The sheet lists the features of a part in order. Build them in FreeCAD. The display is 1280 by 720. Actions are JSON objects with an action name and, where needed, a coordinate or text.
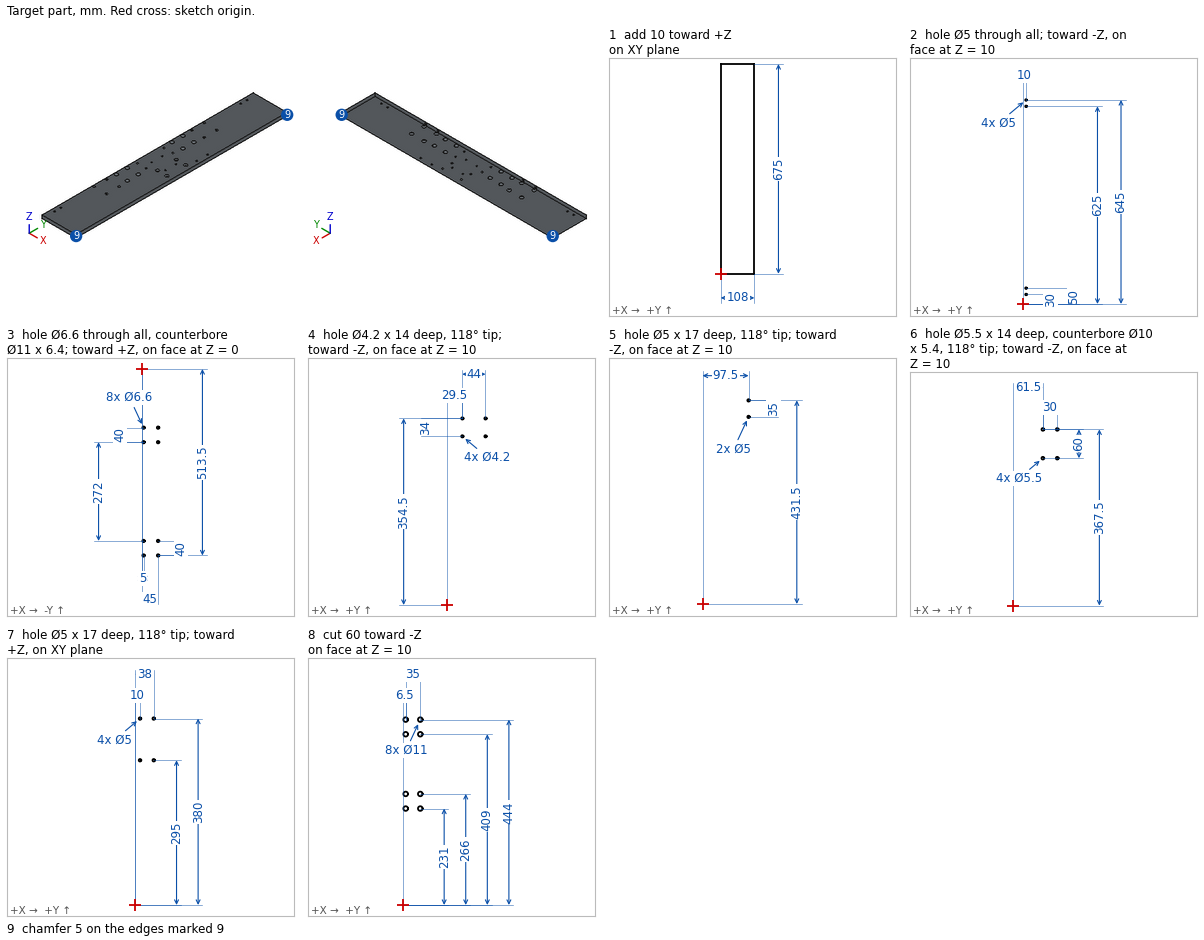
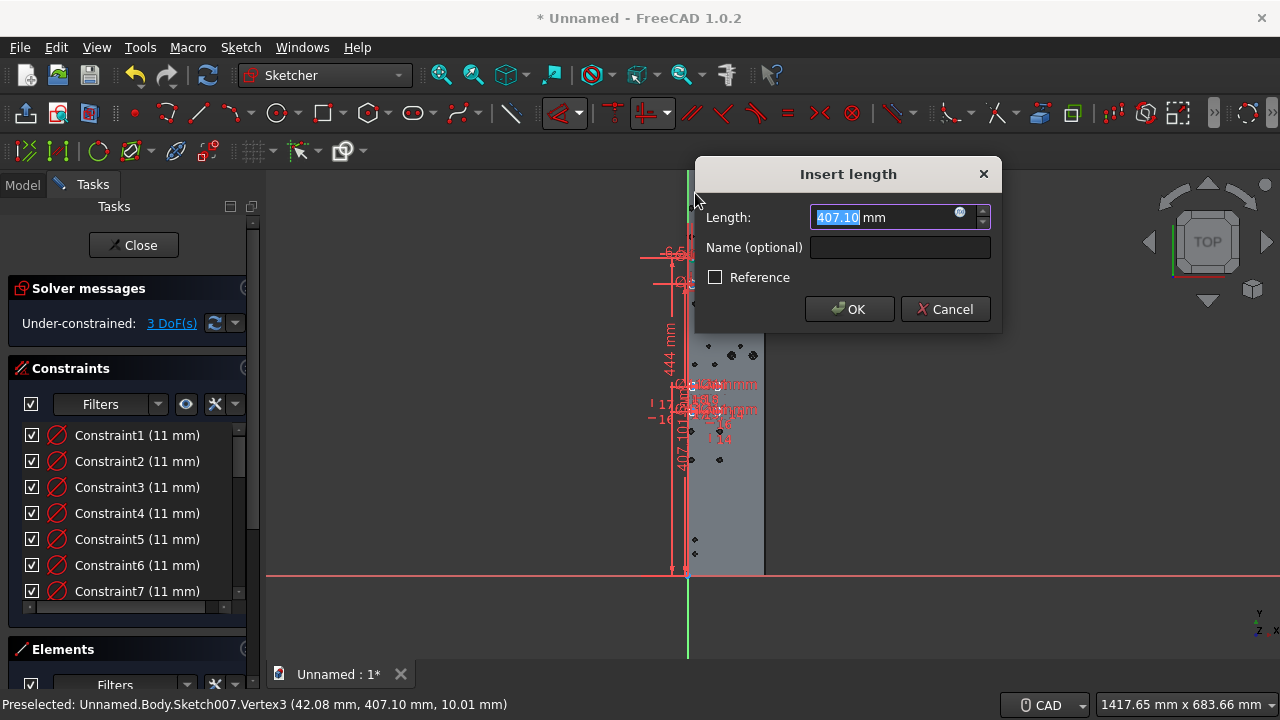
{"action": "type", "text": "409"}
{"action": "key", "text": "Return"}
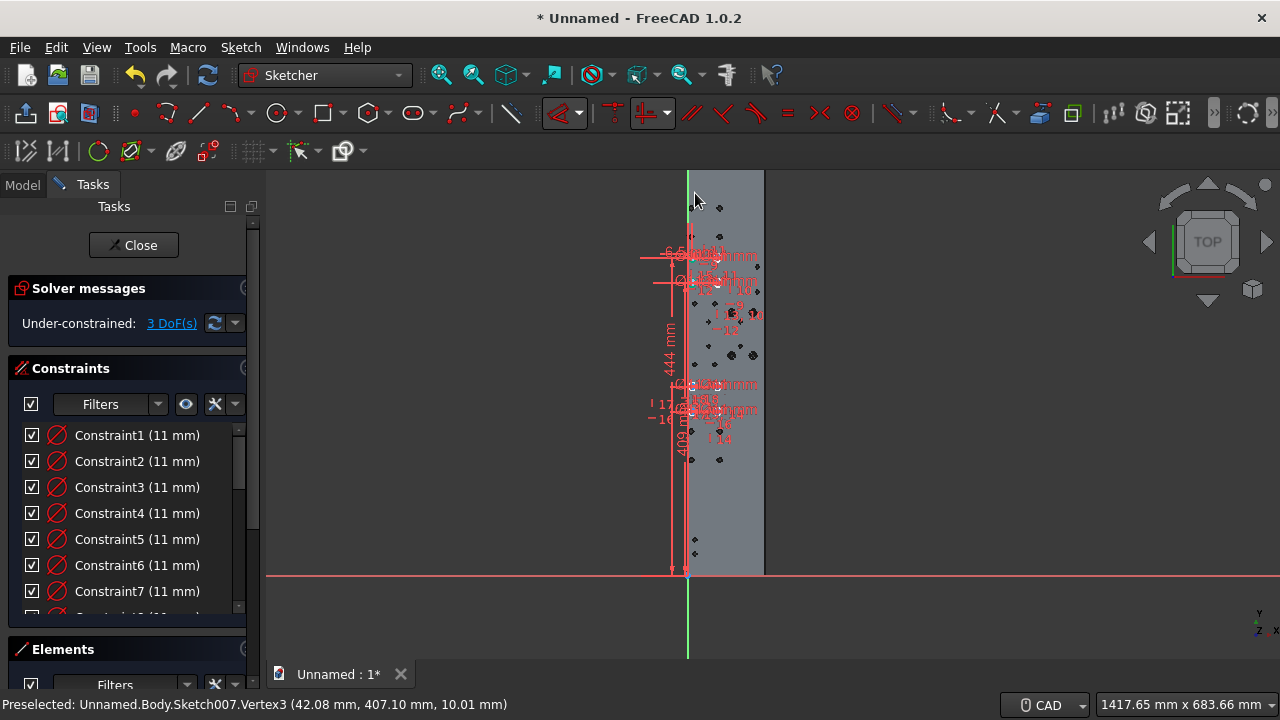
{"action": "left_click", "coordinate": [718, 387]}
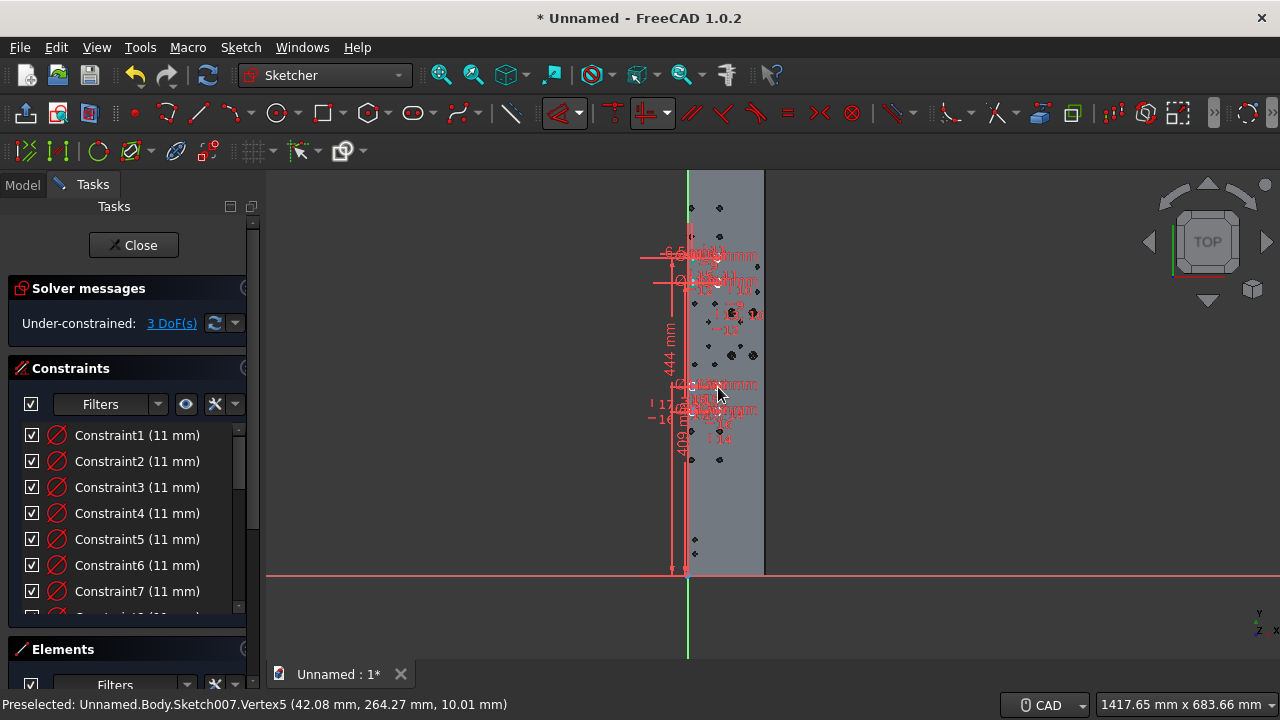
{"action": "left_click", "coordinate": [582, 114]}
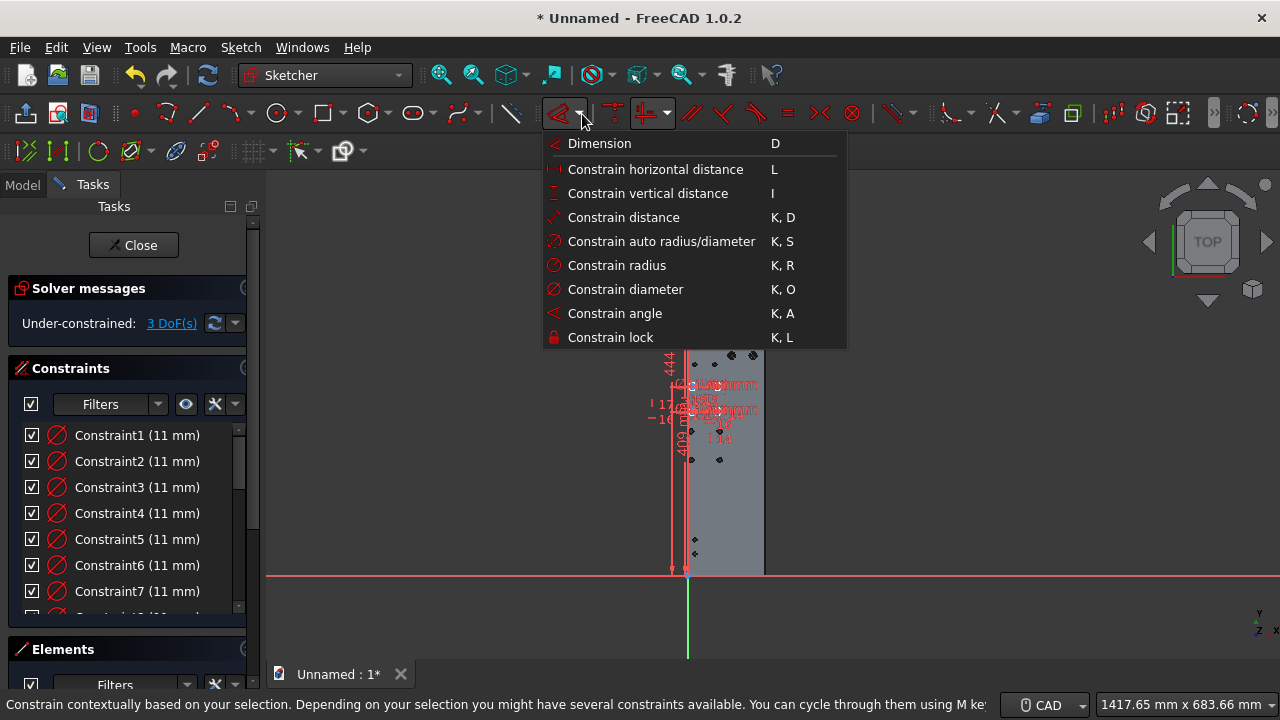
{"action": "left_click", "coordinate": [695, 193]}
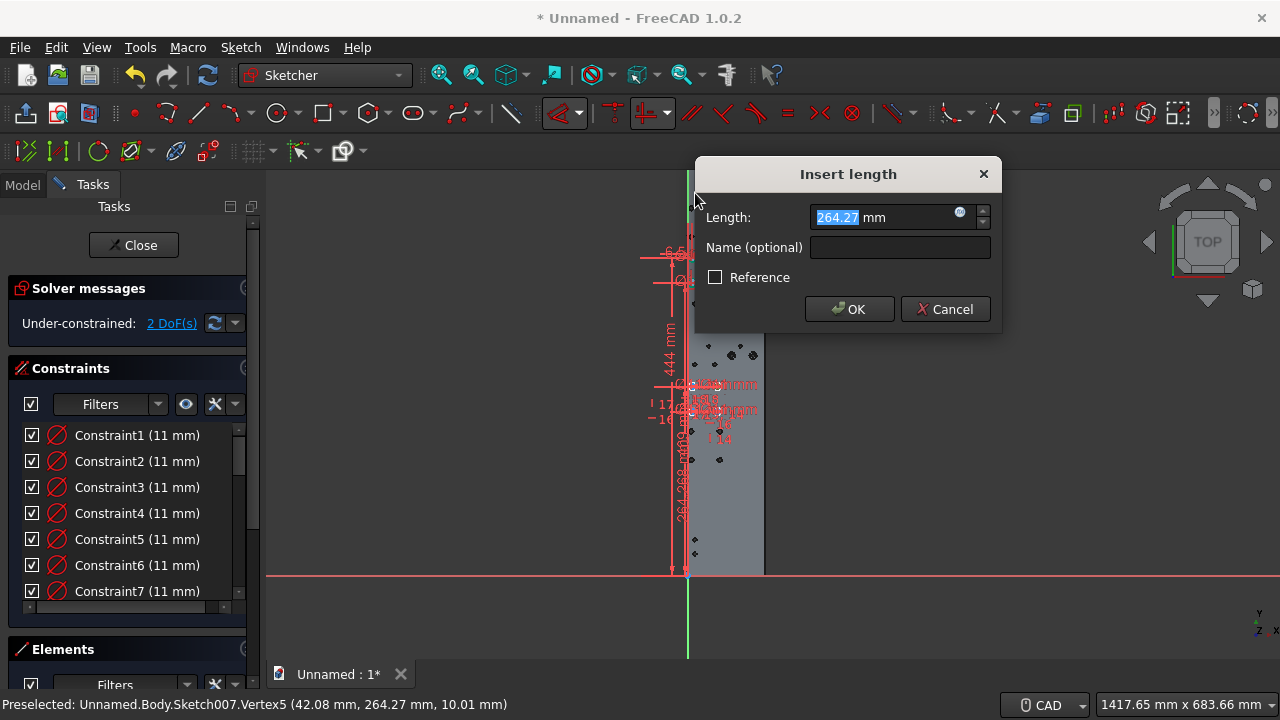
{"action": "type", "text": "266"}
{"action": "key", "text": "Return"}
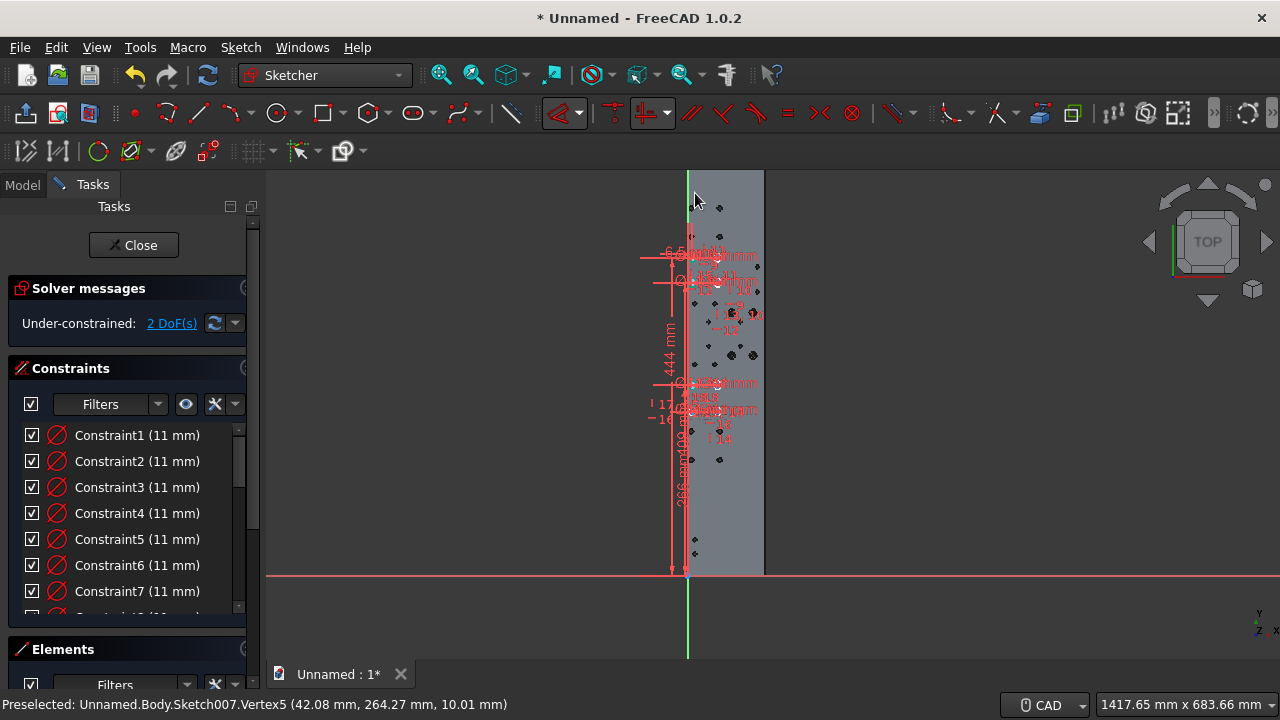
{"action": "left_click", "coordinate": [718, 412]}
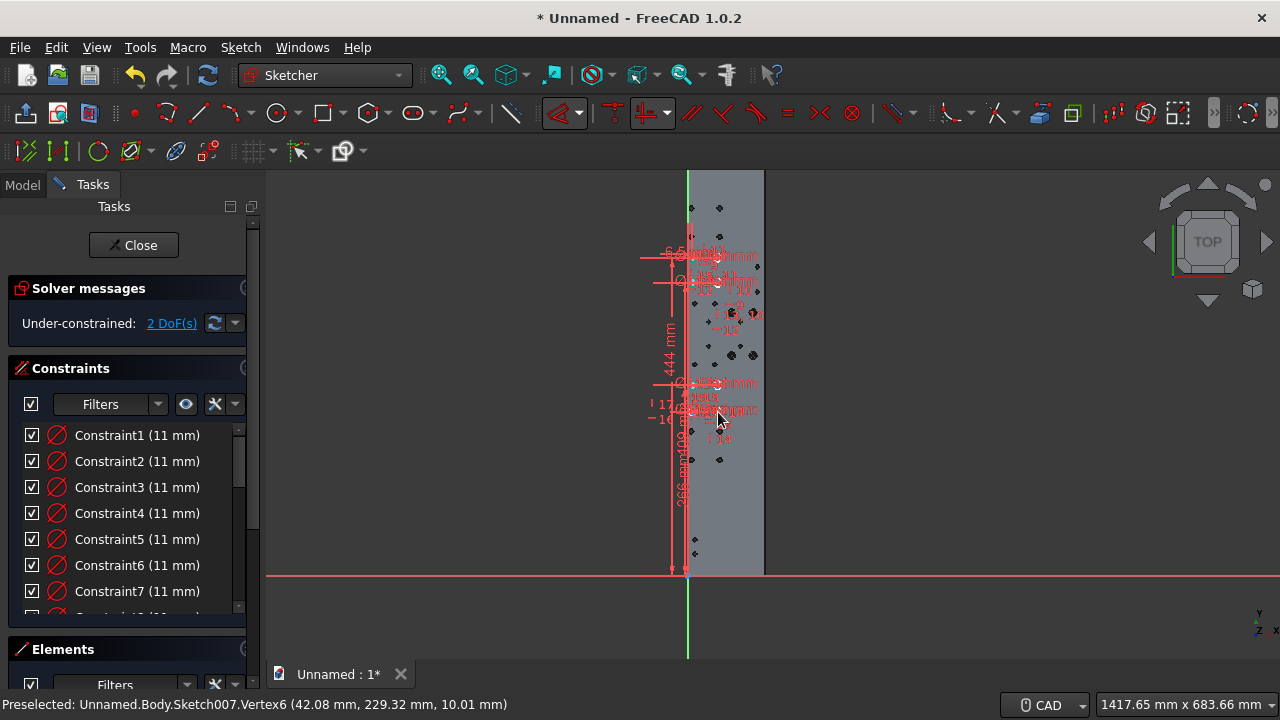
{"action": "key", "text": "i"}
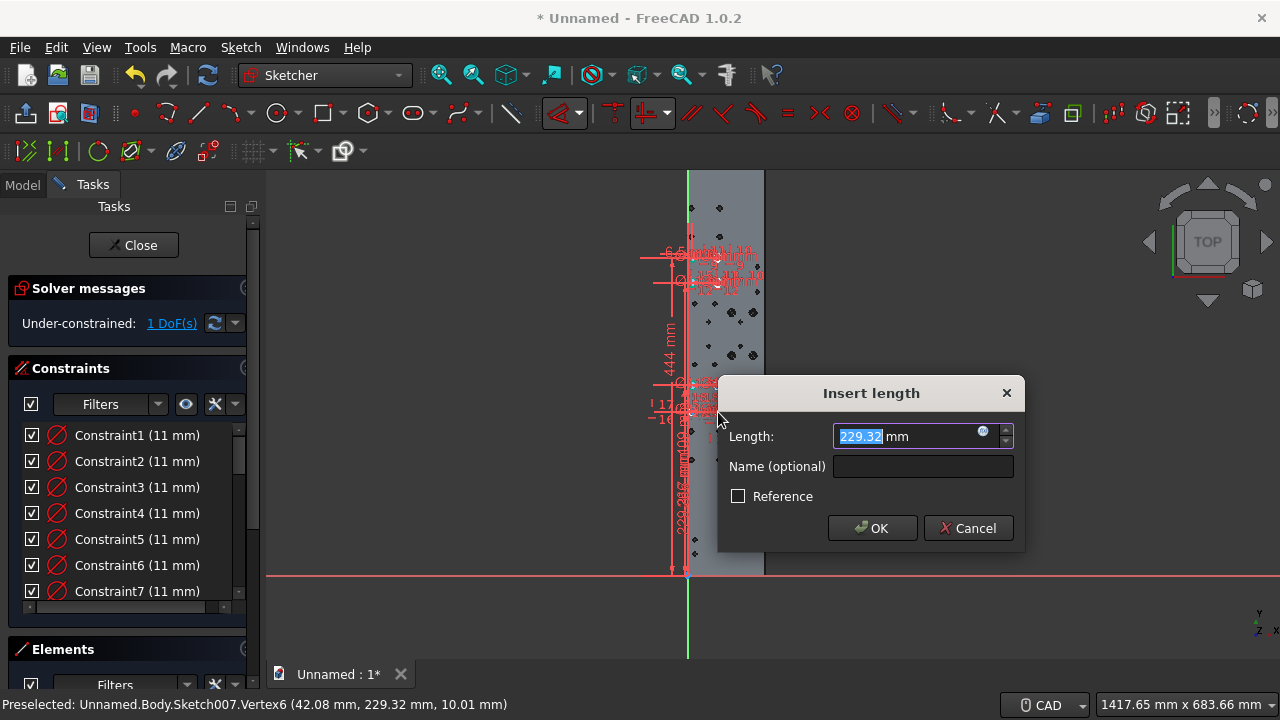
{"action": "type", "text": "231"}
{"action": "key", "text": "Return"}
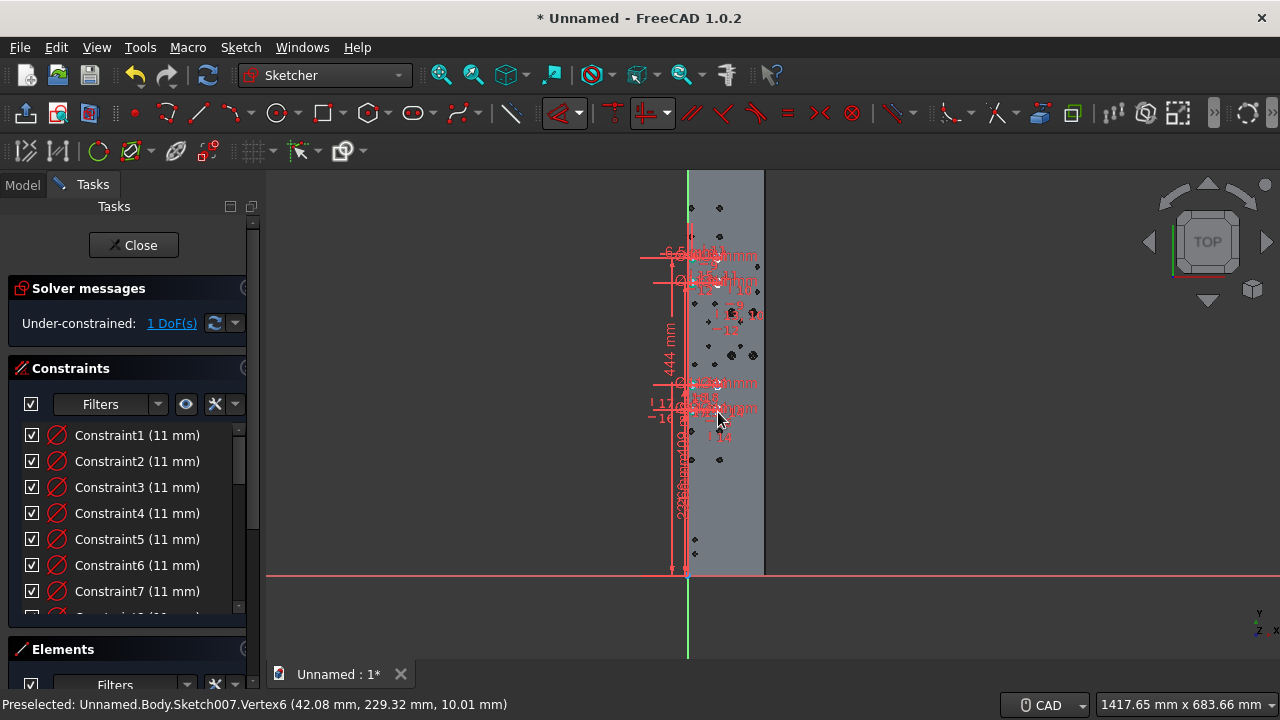
{"action": "scroll", "coordinate": [718, 258], "scroll_direction": "up", "scroll_amount": 3}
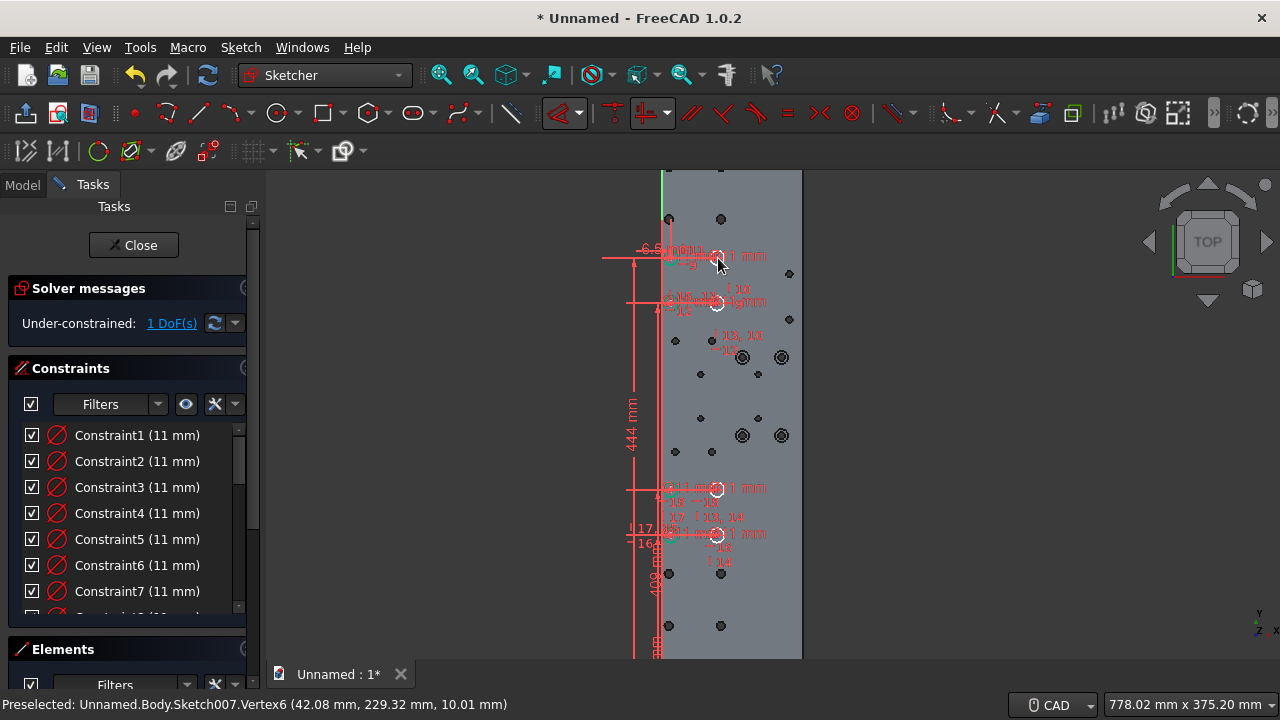
{"action": "left_click", "coordinate": [717, 258]}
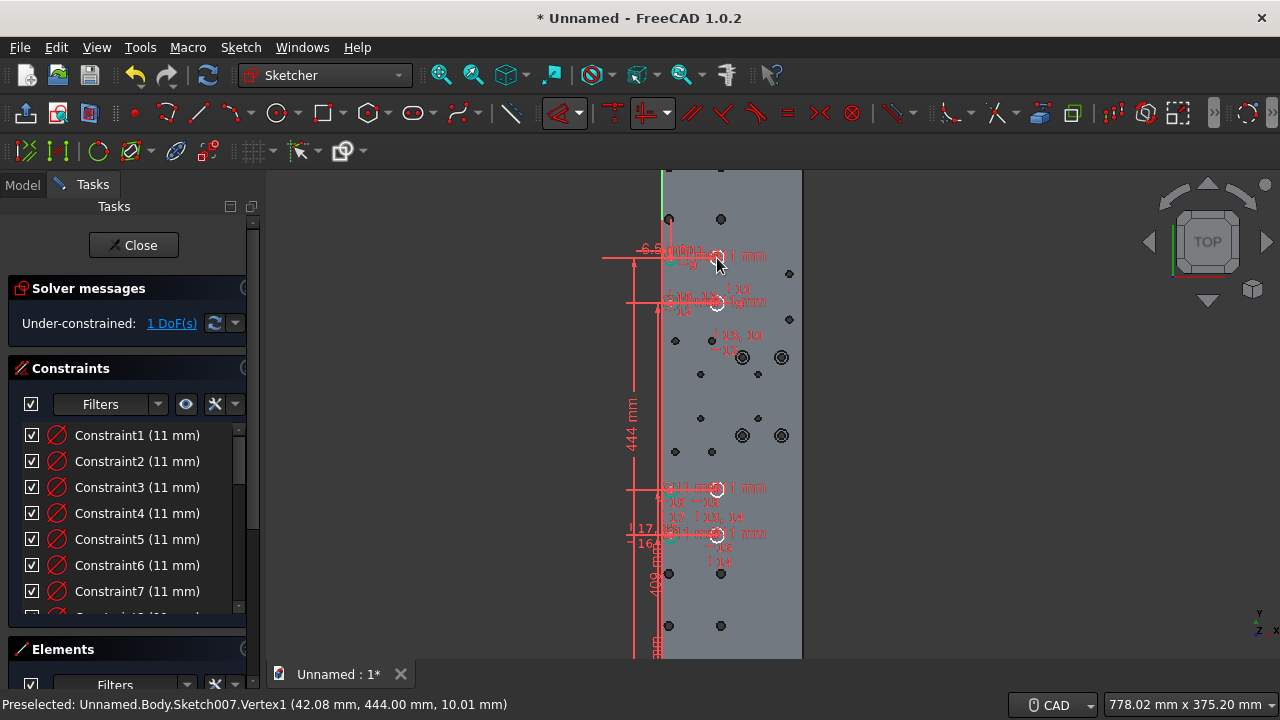
{"action": "left_click", "coordinate": [671, 258]}